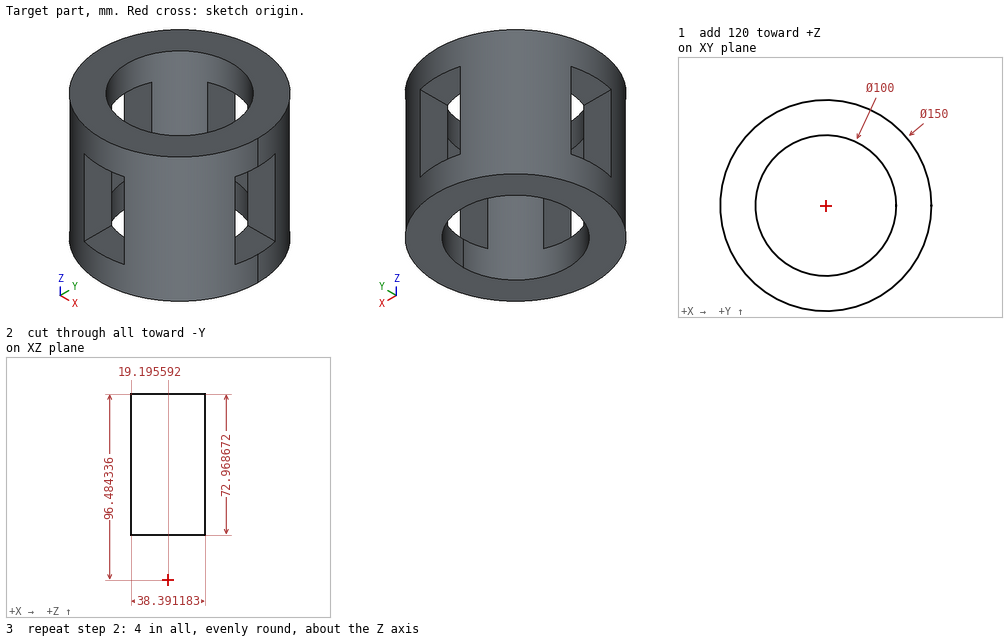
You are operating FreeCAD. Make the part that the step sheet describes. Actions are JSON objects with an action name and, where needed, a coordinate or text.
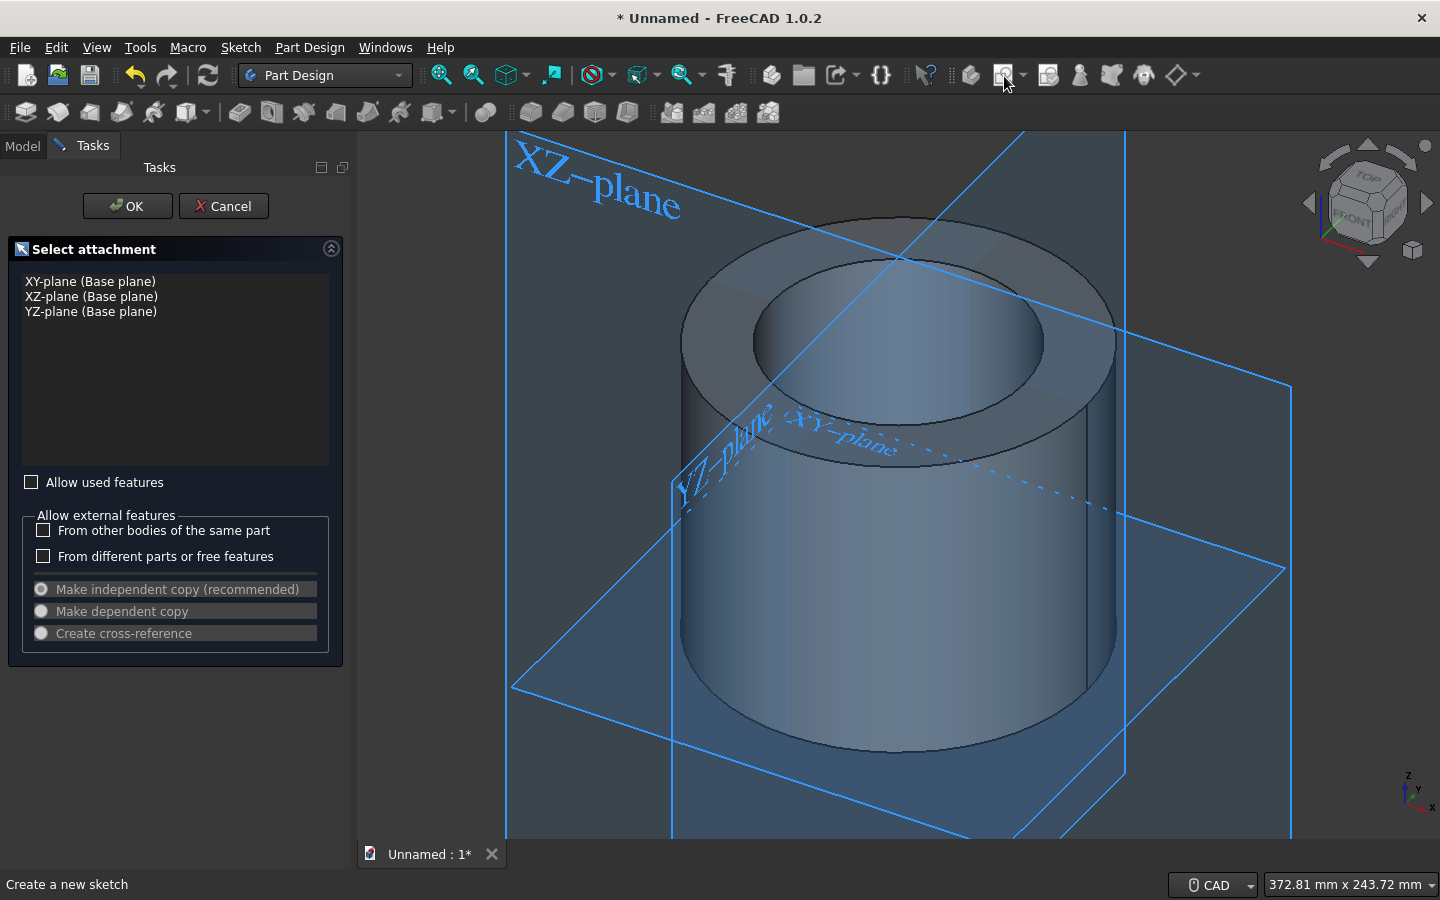
{"action": "left_click", "coordinate": [82, 296]}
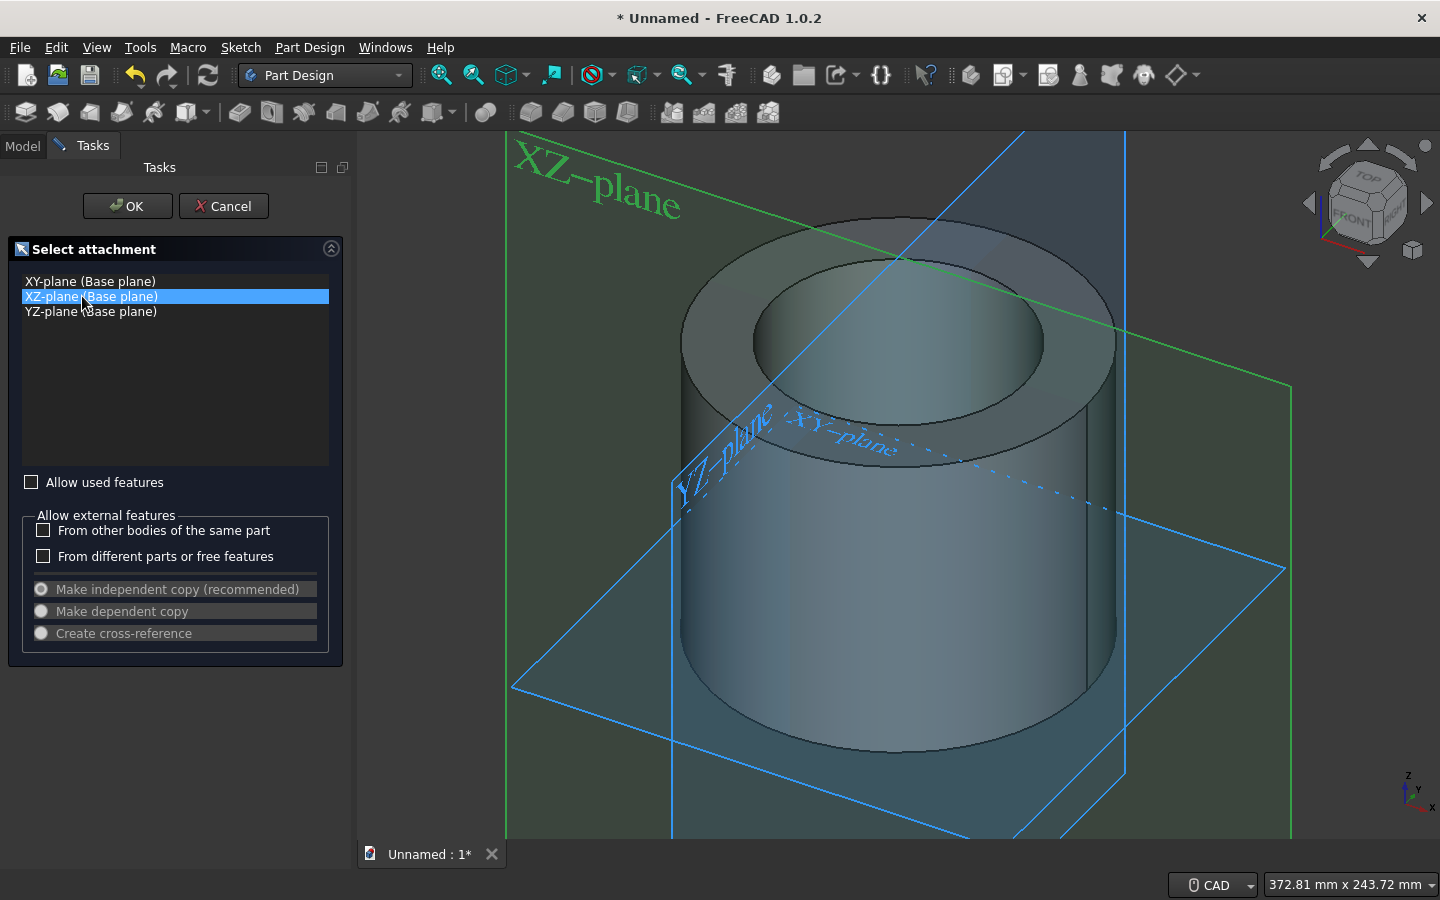
{"action": "left_click", "coordinate": [128, 206]}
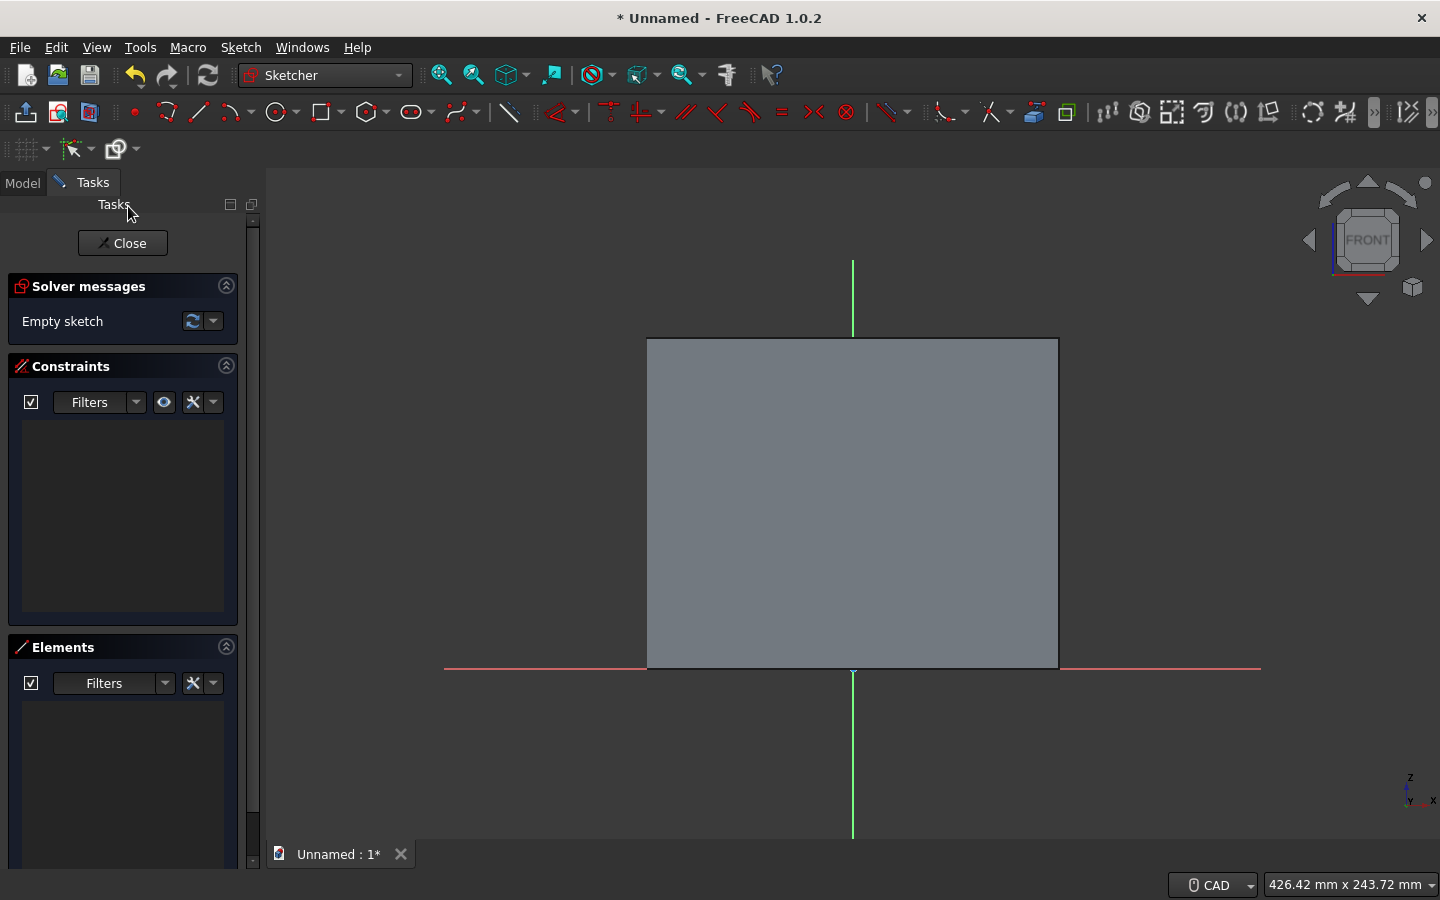
{"action": "left_click", "coordinate": [90, 112]}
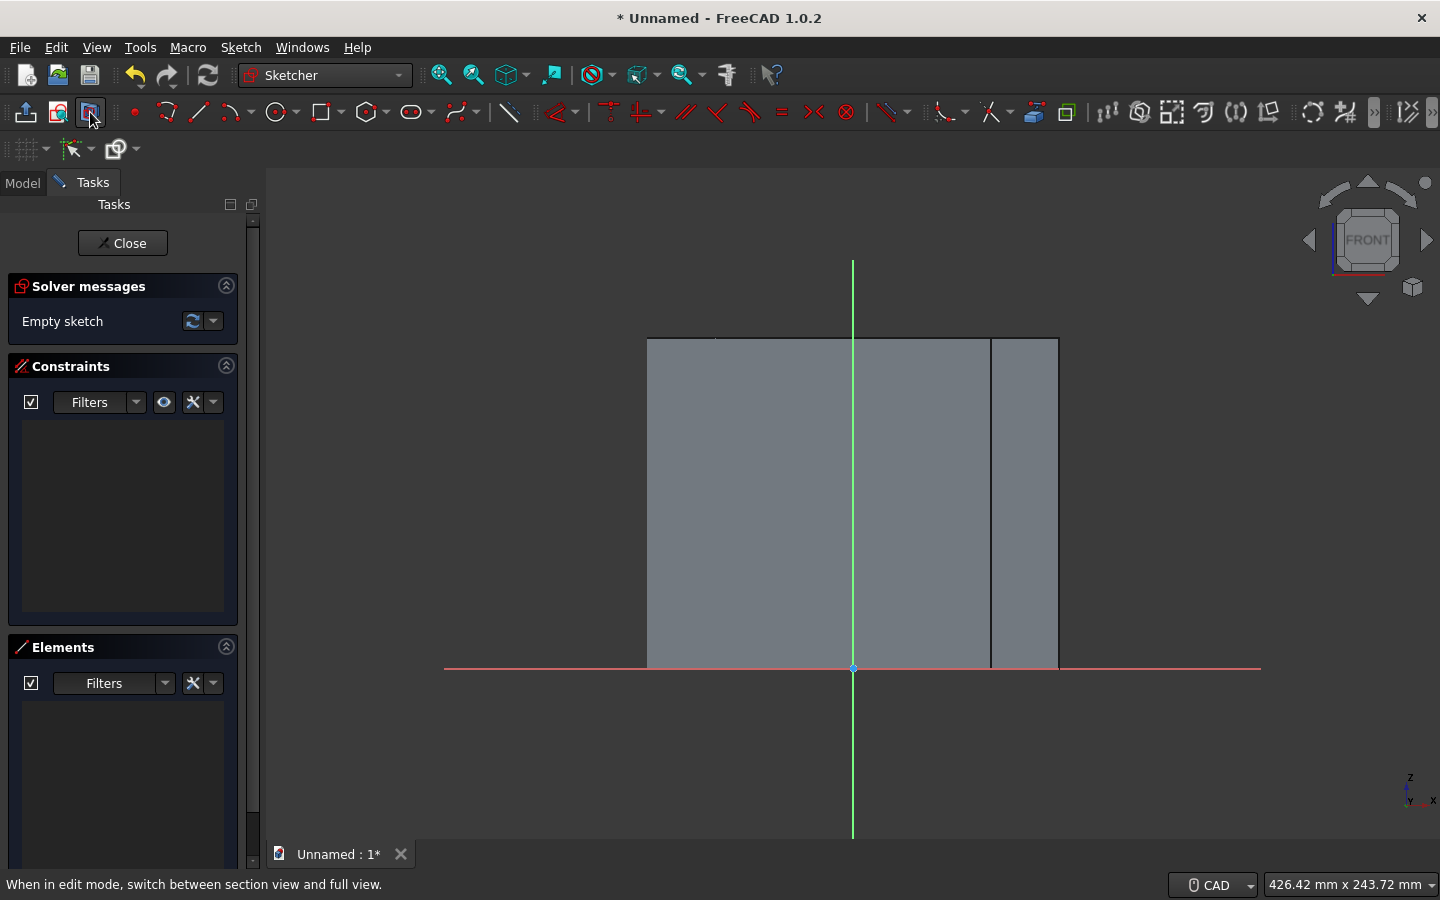
{"action": "scroll", "coordinate": [992, 602], "scroll_direction": "up", "scroll_amount": 2}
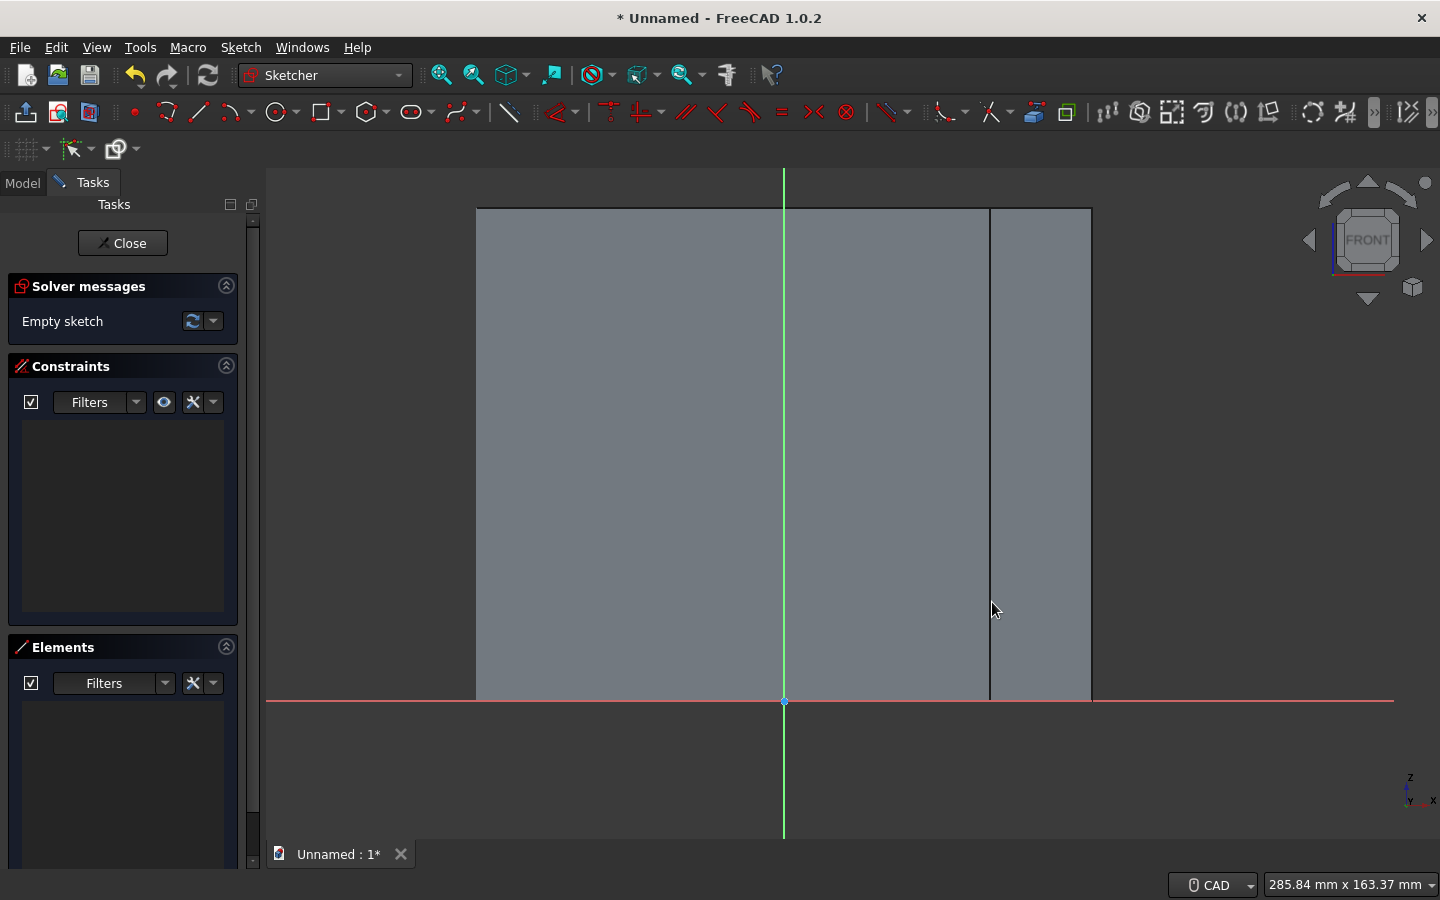
{"action": "left_click", "coordinate": [322, 112]}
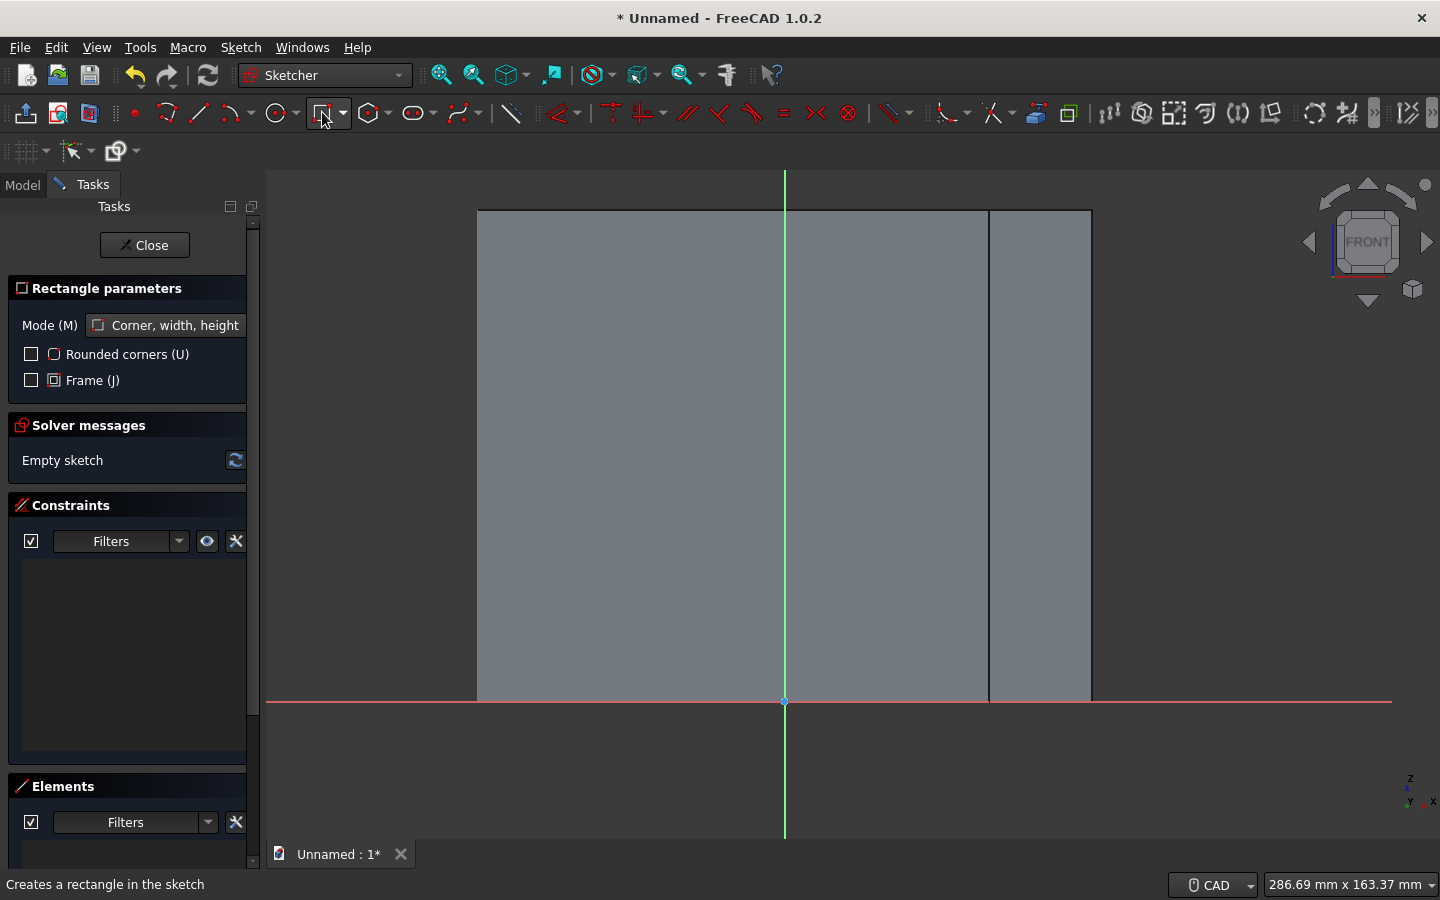
{"action": "left_click", "coordinate": [706, 306]}
{"action": "mouse_move", "coordinate": [863, 605]}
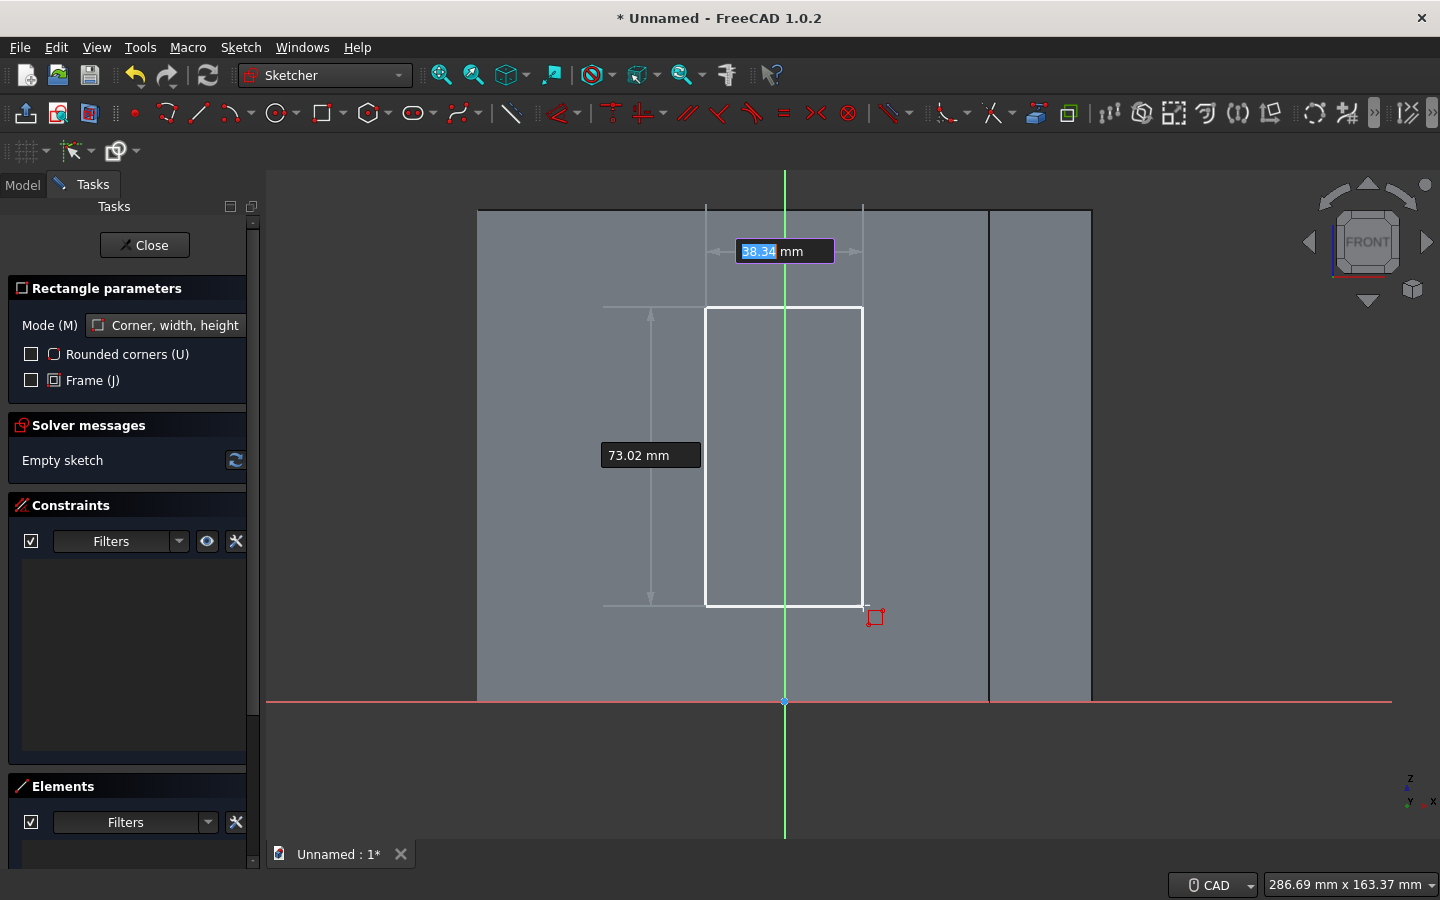
{"action": "type", "text": "38.391183"}
{"action": "key", "text": "Tab"}
{"action": "type", "text": "72.968672"}
{"action": "key", "text": "Return"}
{"action": "key", "text": "Escape"}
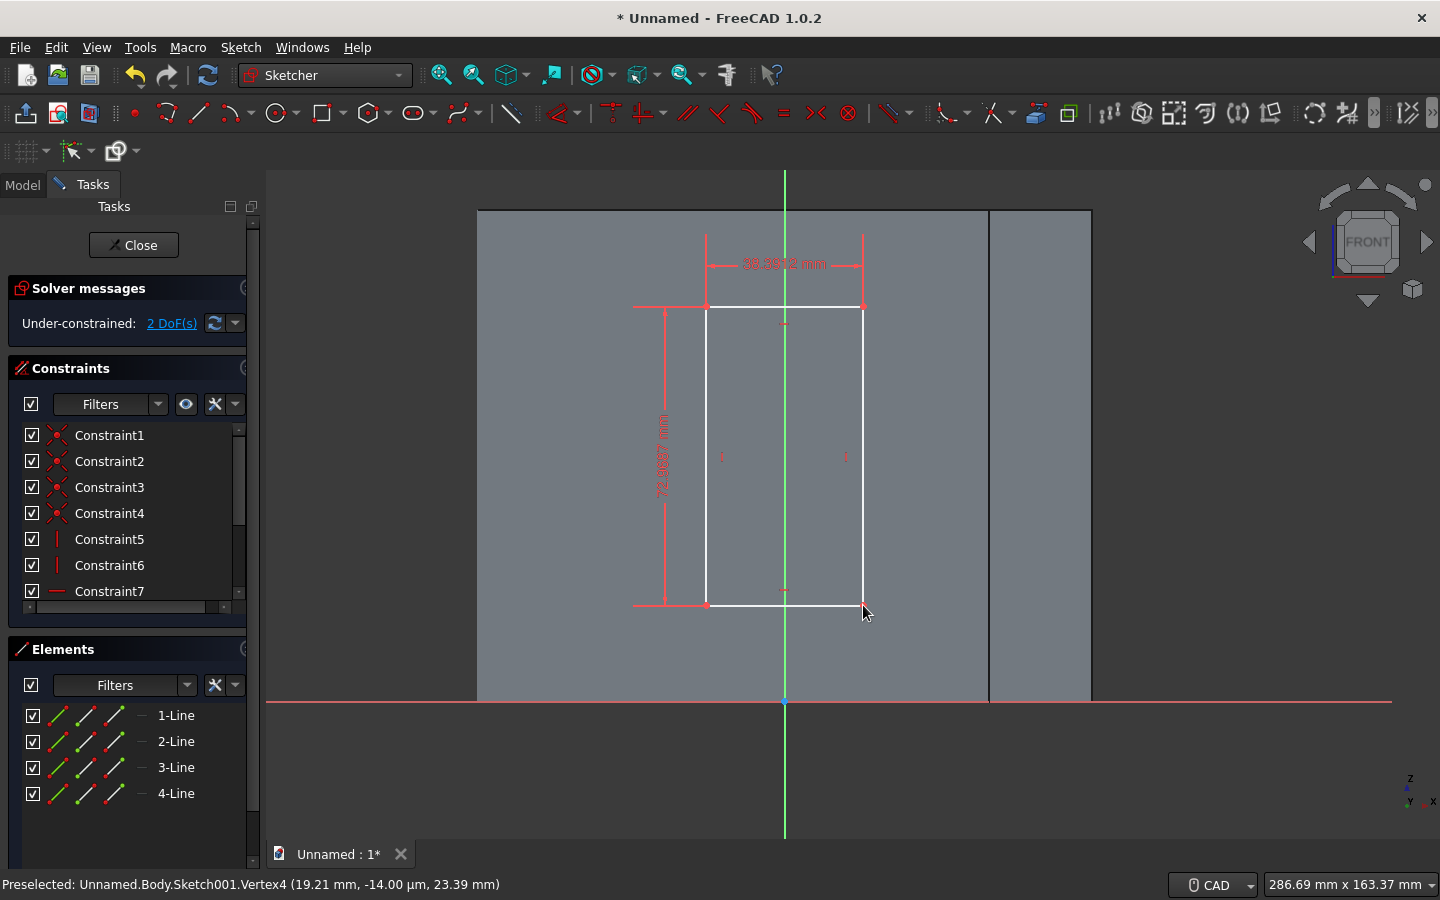
{"action": "left_click", "coordinate": [558, 114]}